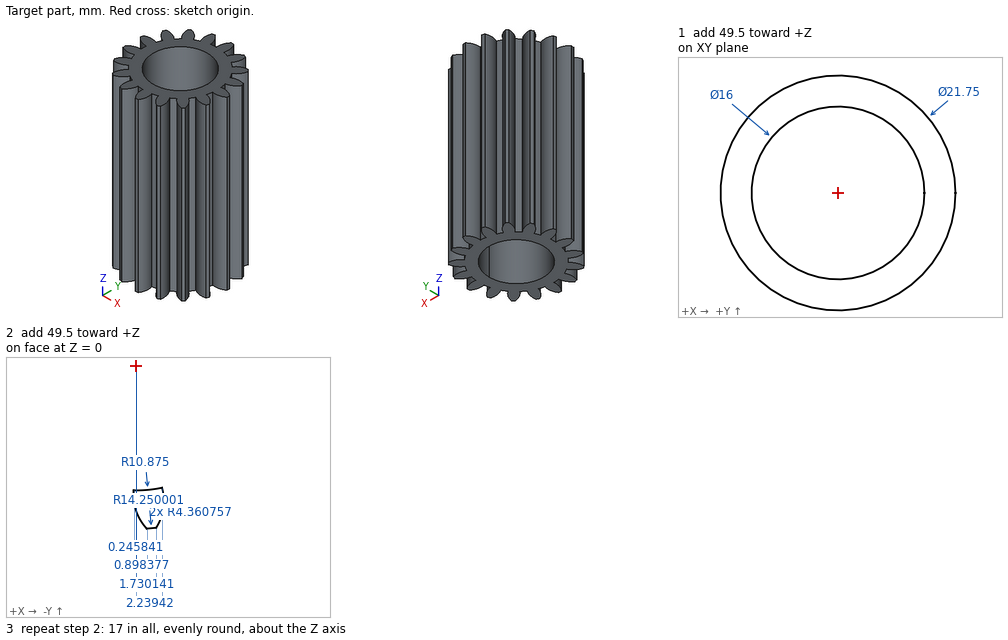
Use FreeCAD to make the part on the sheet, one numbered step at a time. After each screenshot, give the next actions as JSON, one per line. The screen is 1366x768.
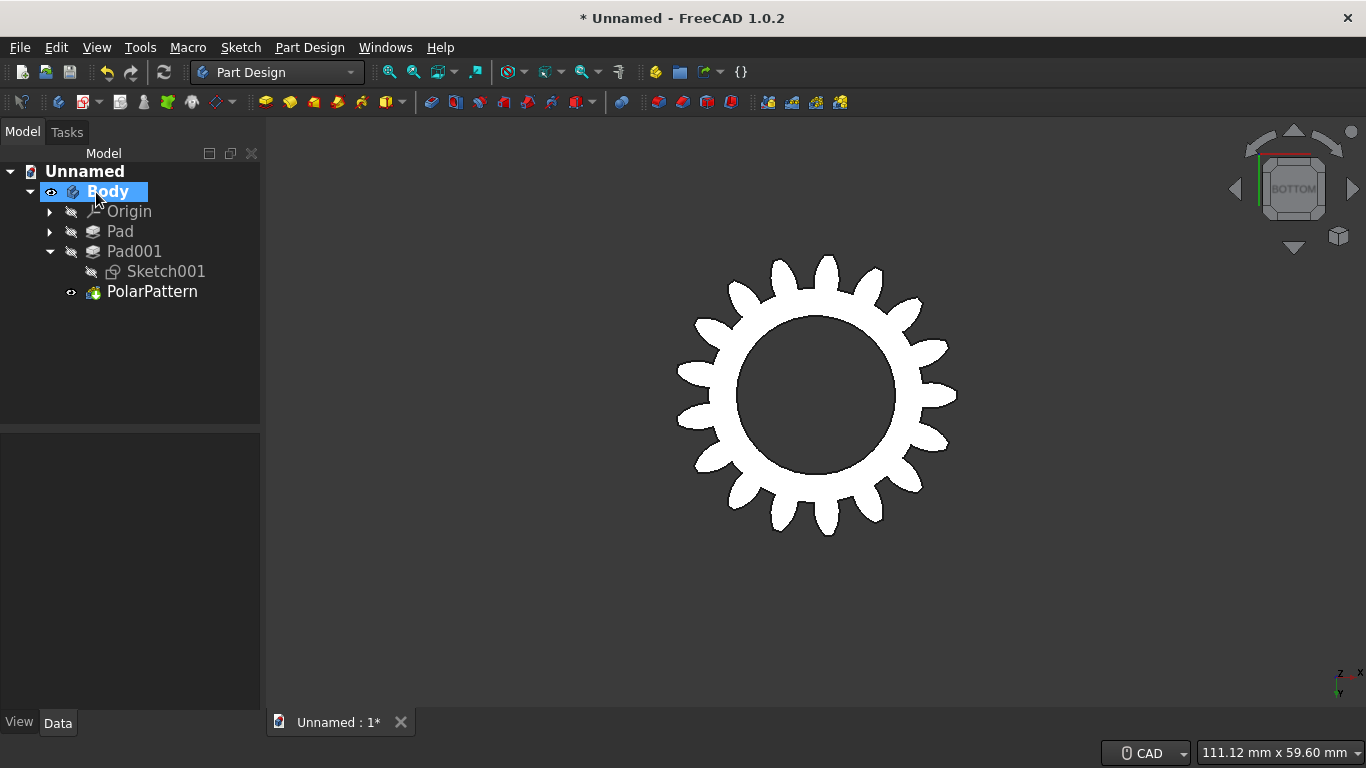
{"action": "key", "text": "0"}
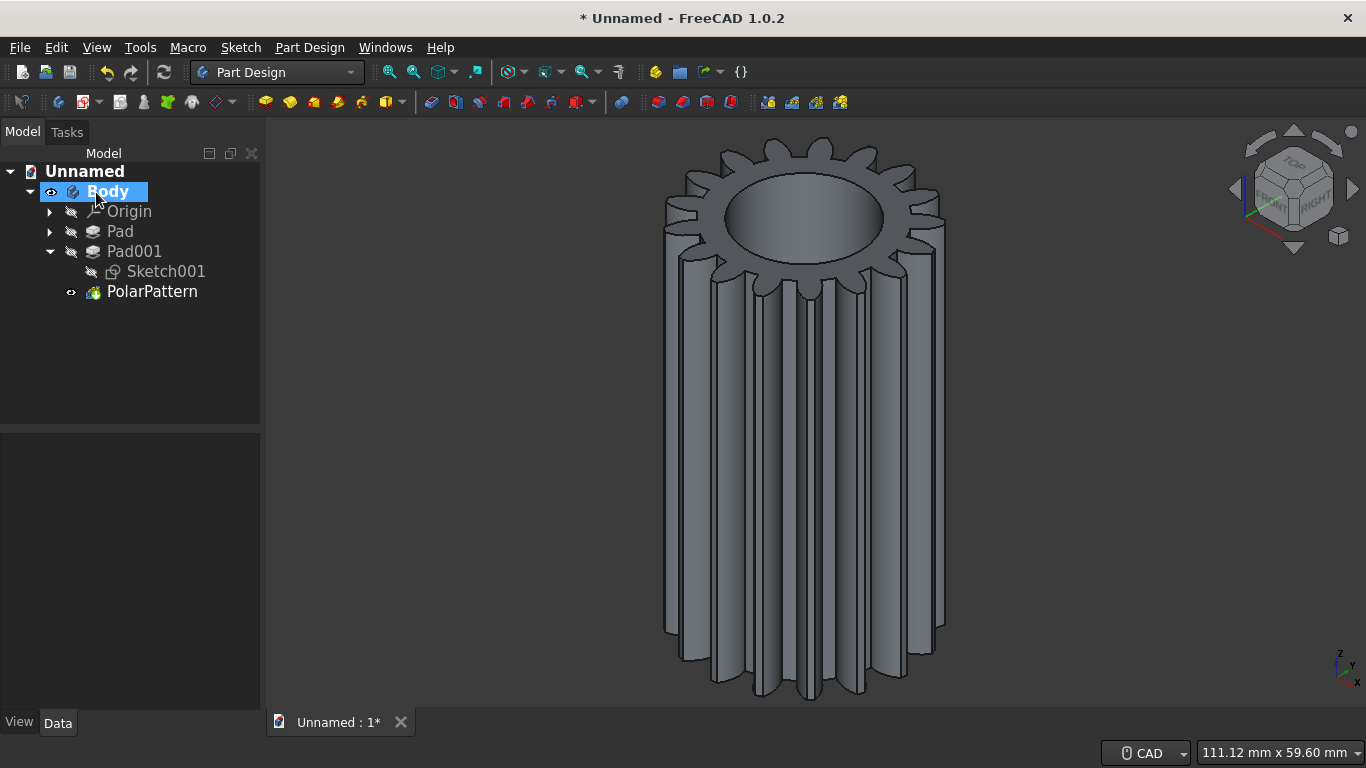
{"action": "left_click", "coordinate": [390, 72]}